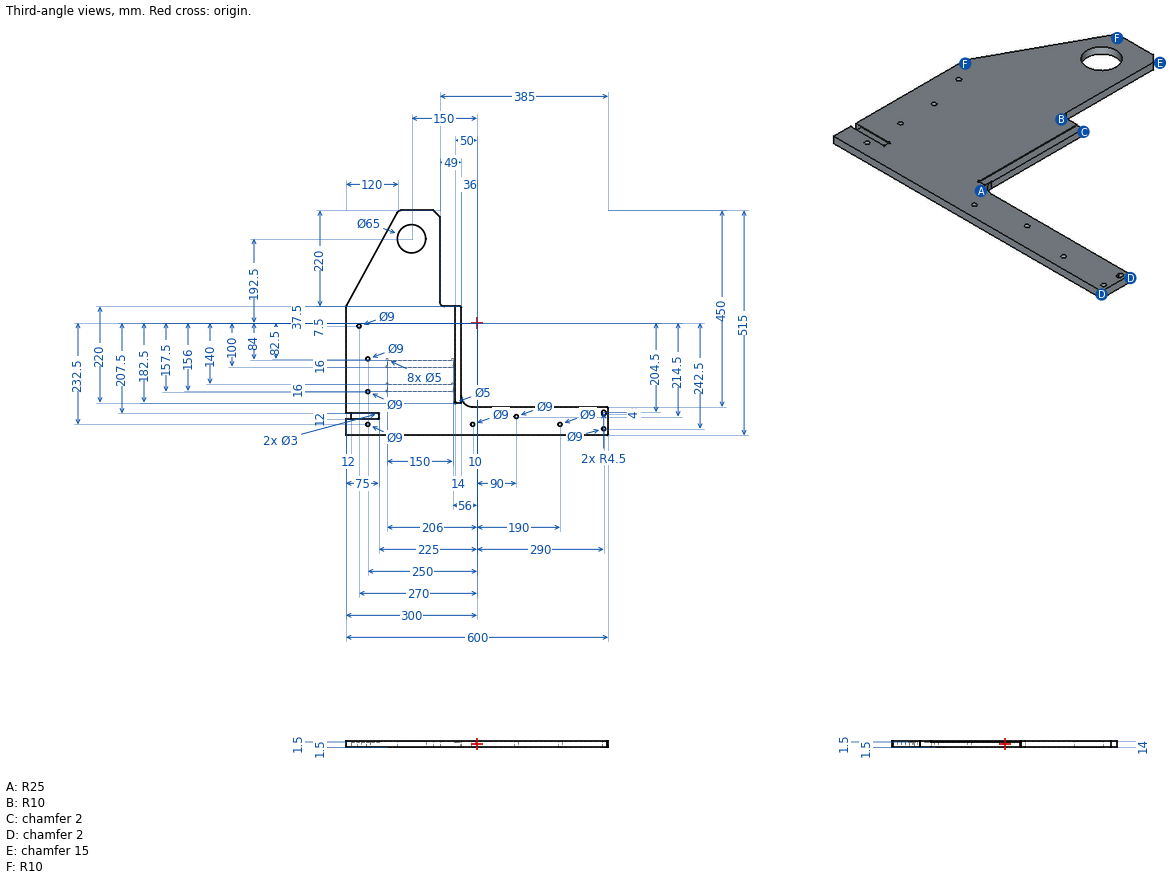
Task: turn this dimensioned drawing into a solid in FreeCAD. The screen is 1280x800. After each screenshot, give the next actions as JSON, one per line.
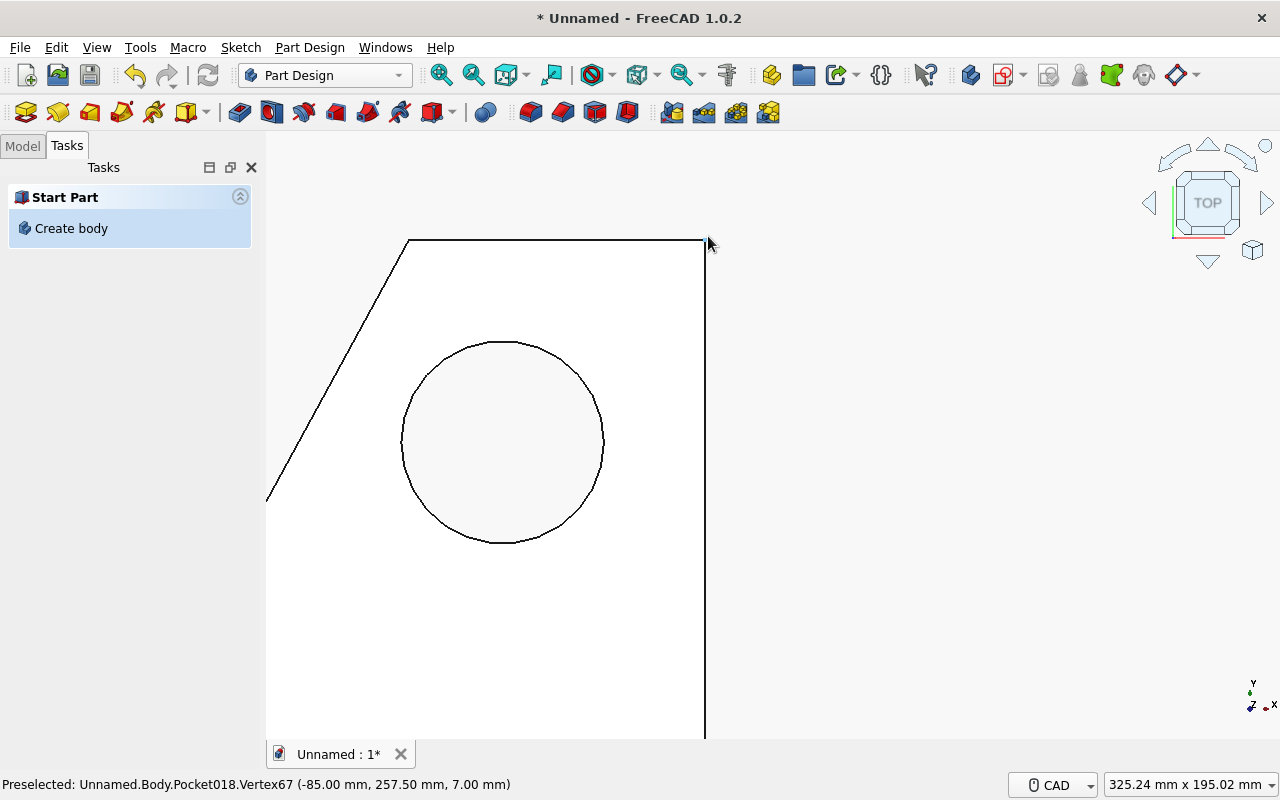
{"action": "left_click", "coordinate": [442, 76]}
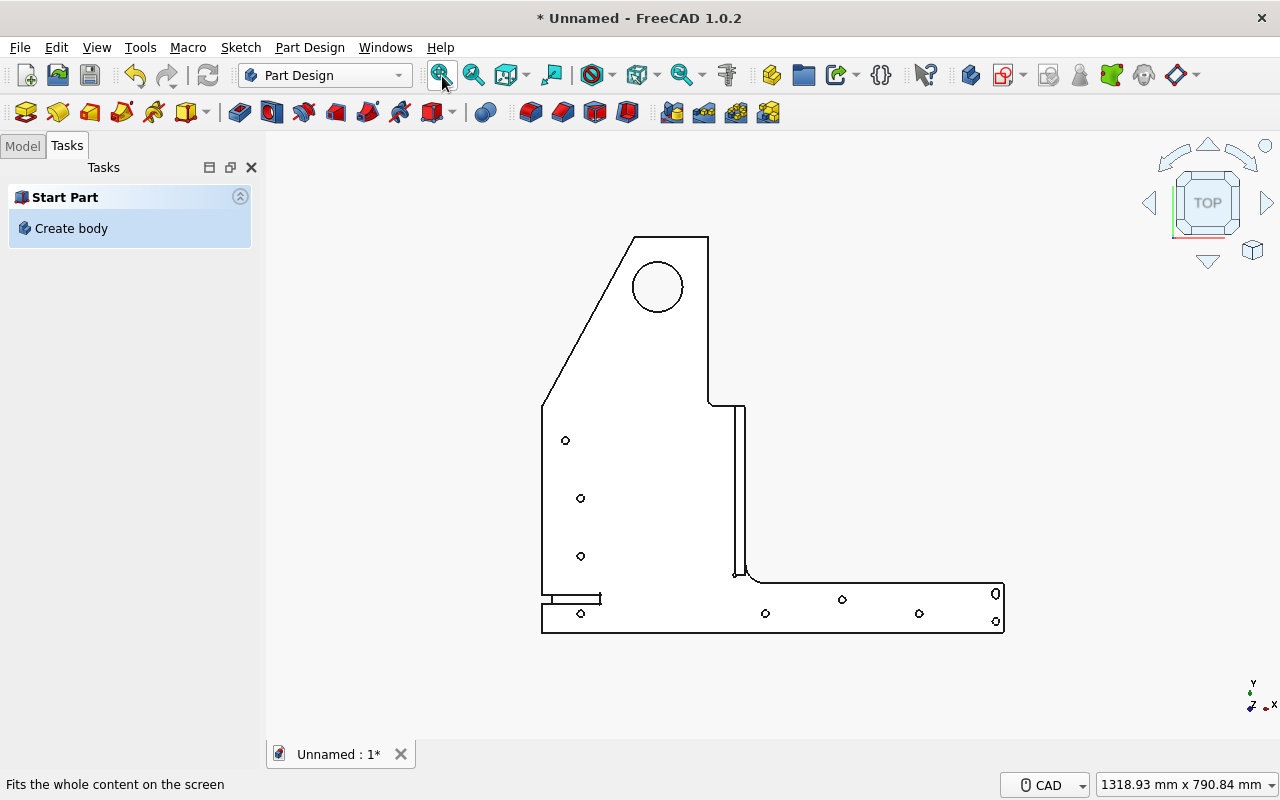
{"action": "key", "text": "0"}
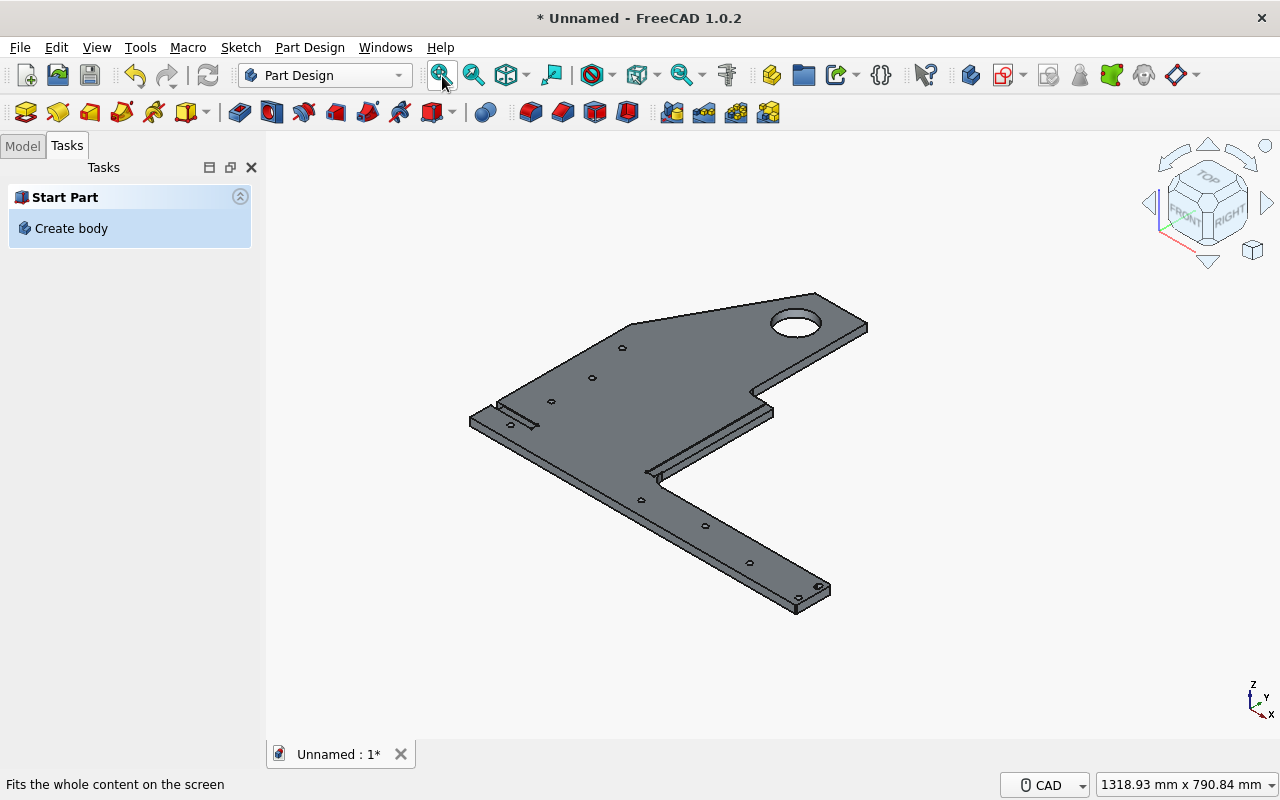
{"action": "scroll", "coordinate": [867, 327], "scroll_direction": "up", "scroll_amount": 7}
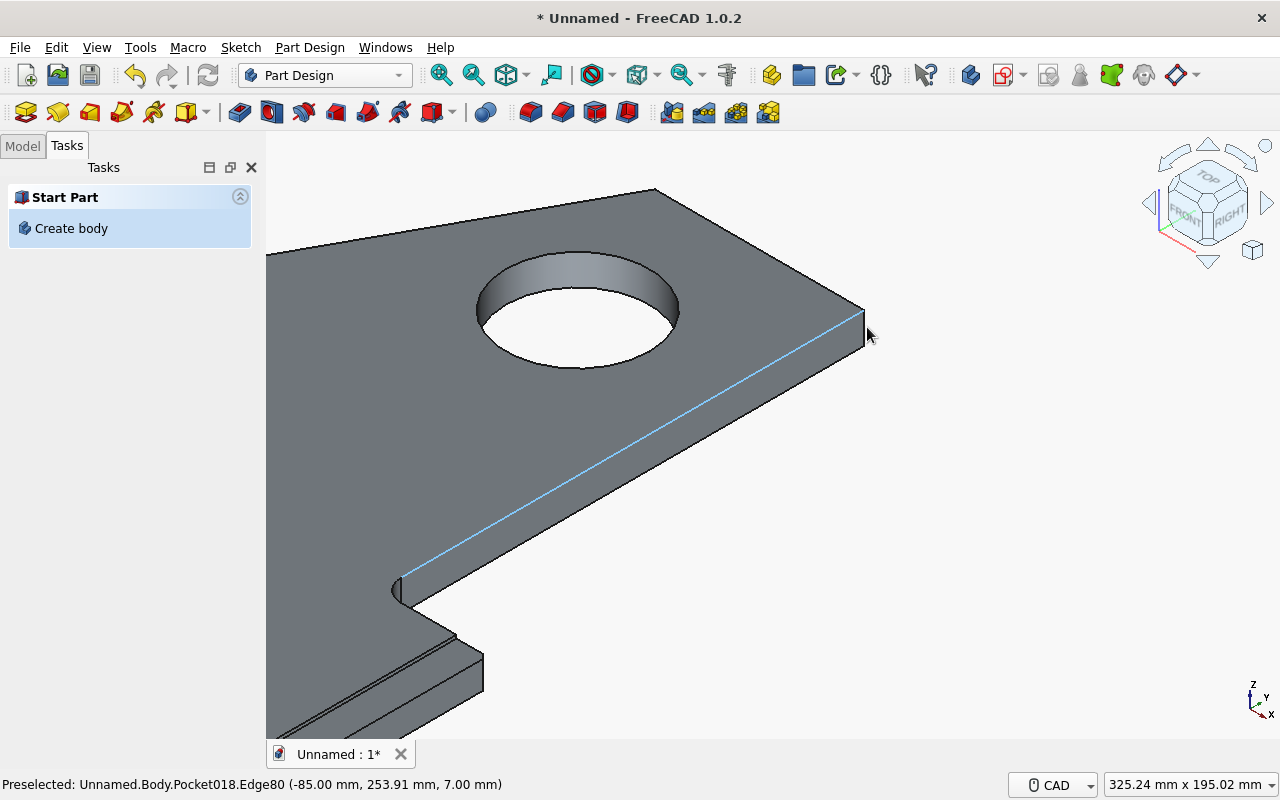
{"action": "left_click", "coordinate": [442, 76]}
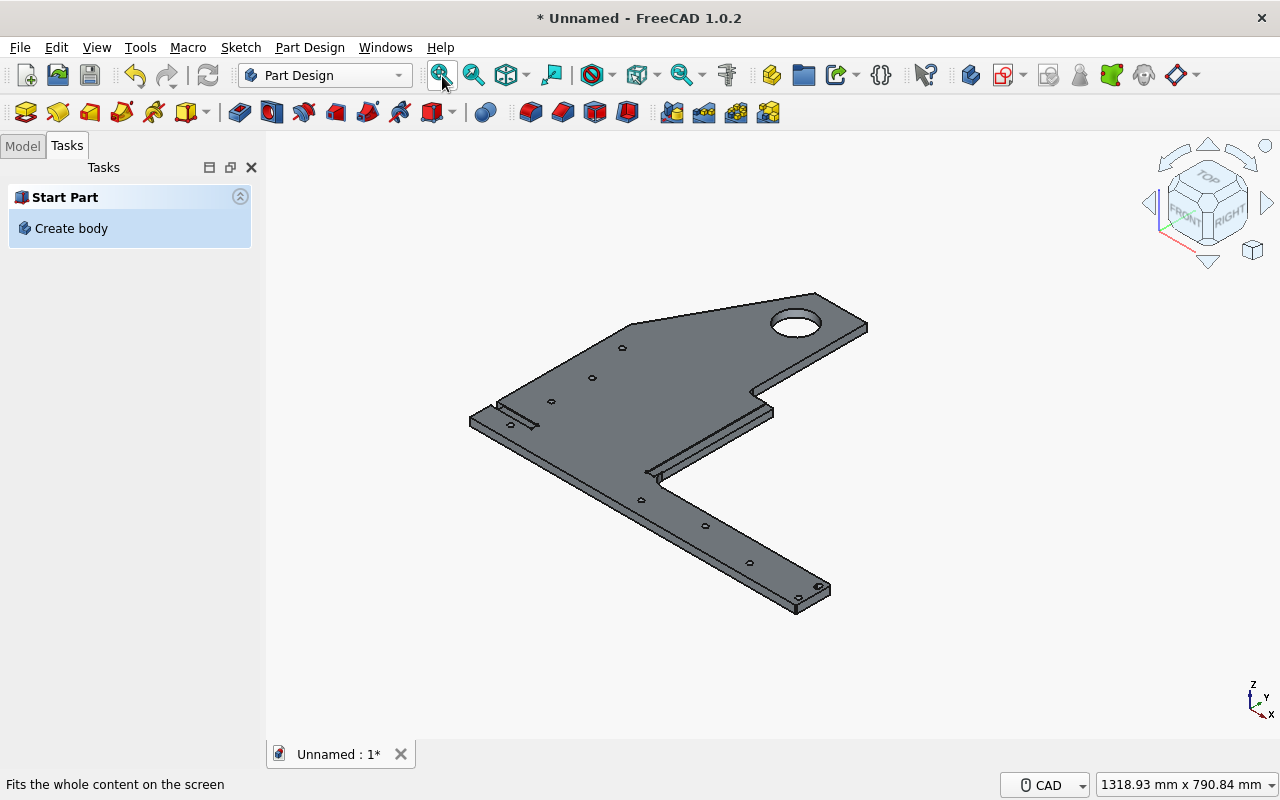
{"action": "key", "text": "1"}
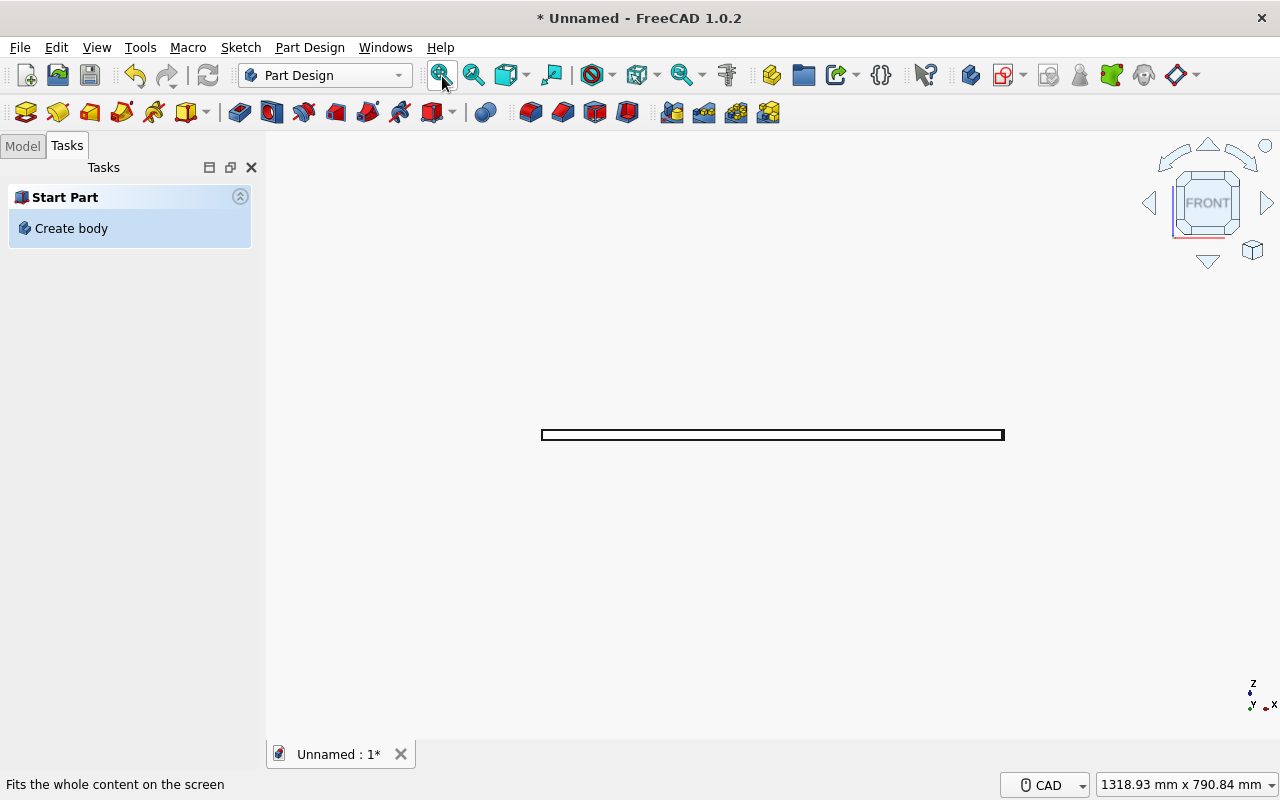
{"action": "scroll", "coordinate": [708, 434], "scroll_direction": "up", "scroll_amount": 7}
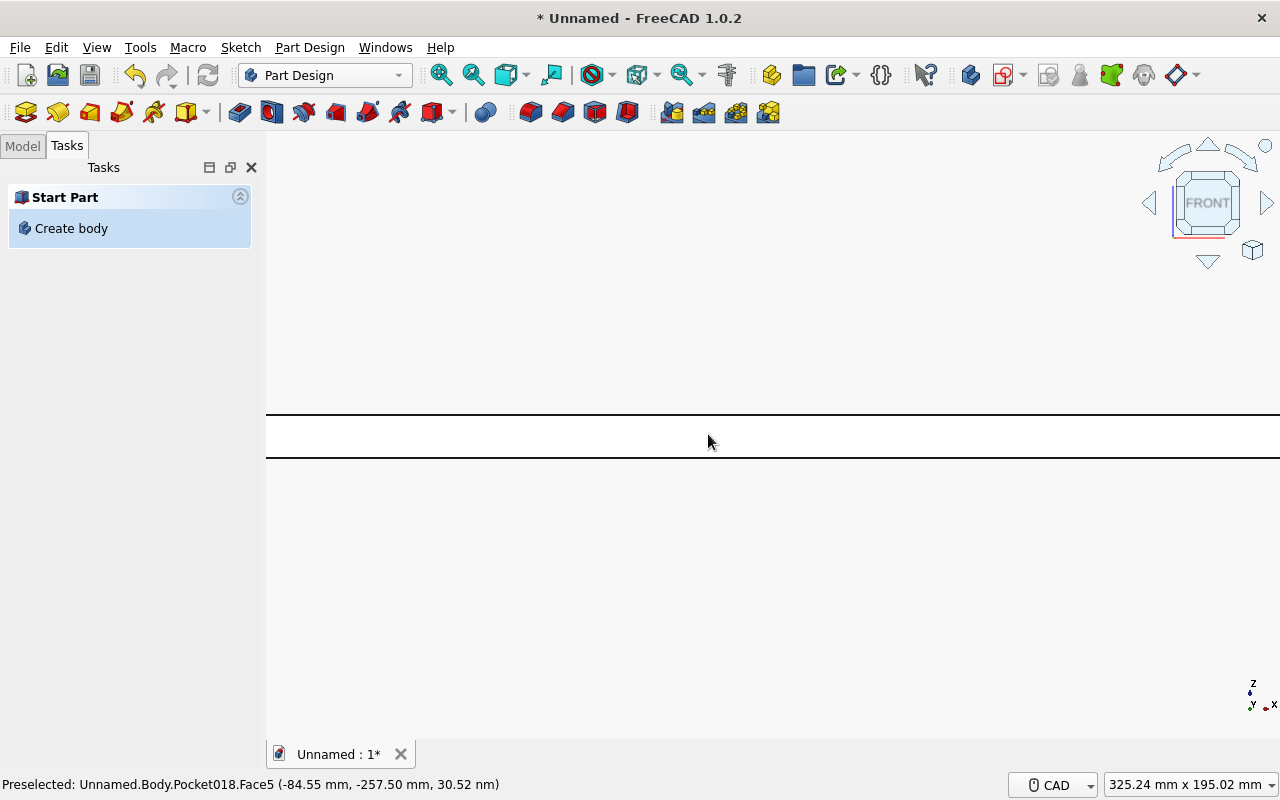
{"action": "left_click", "coordinate": [442, 76]}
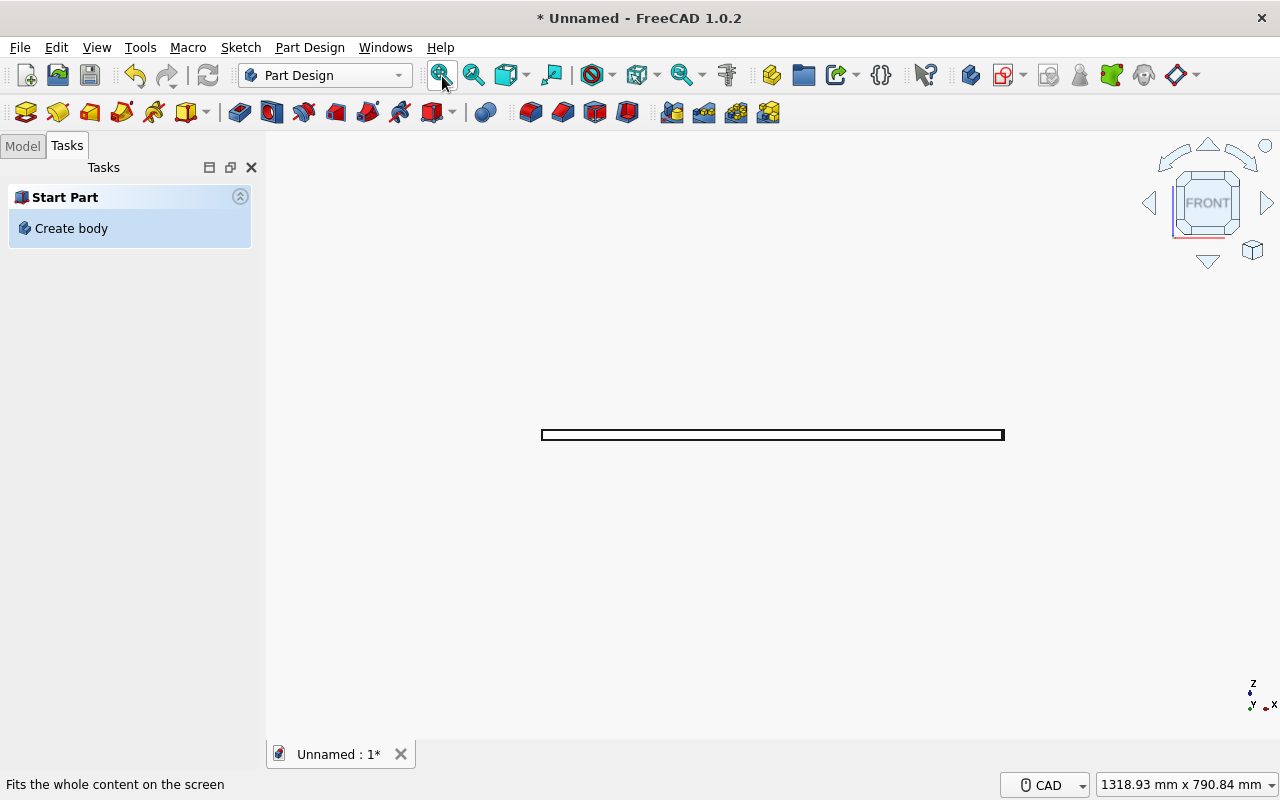
{"action": "key", "text": "3"}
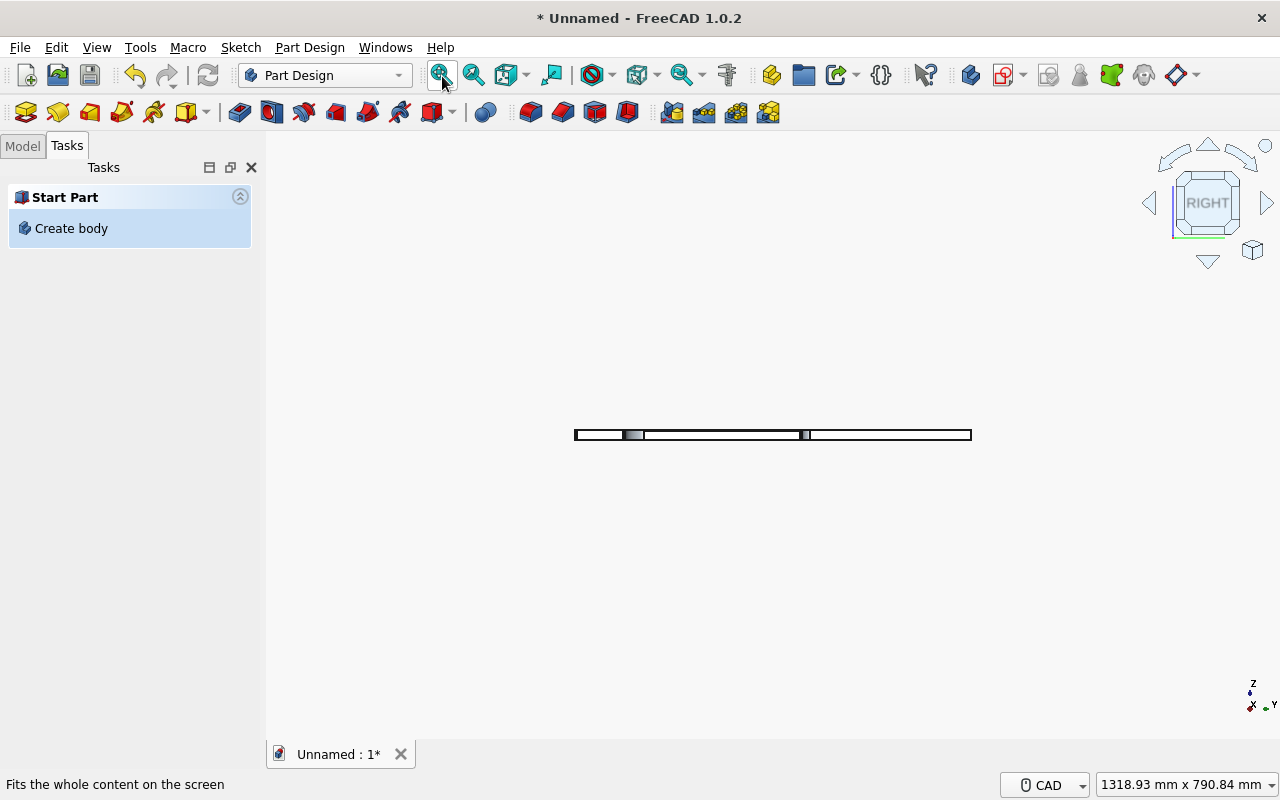
{"action": "left_click", "coordinate": [442, 76]}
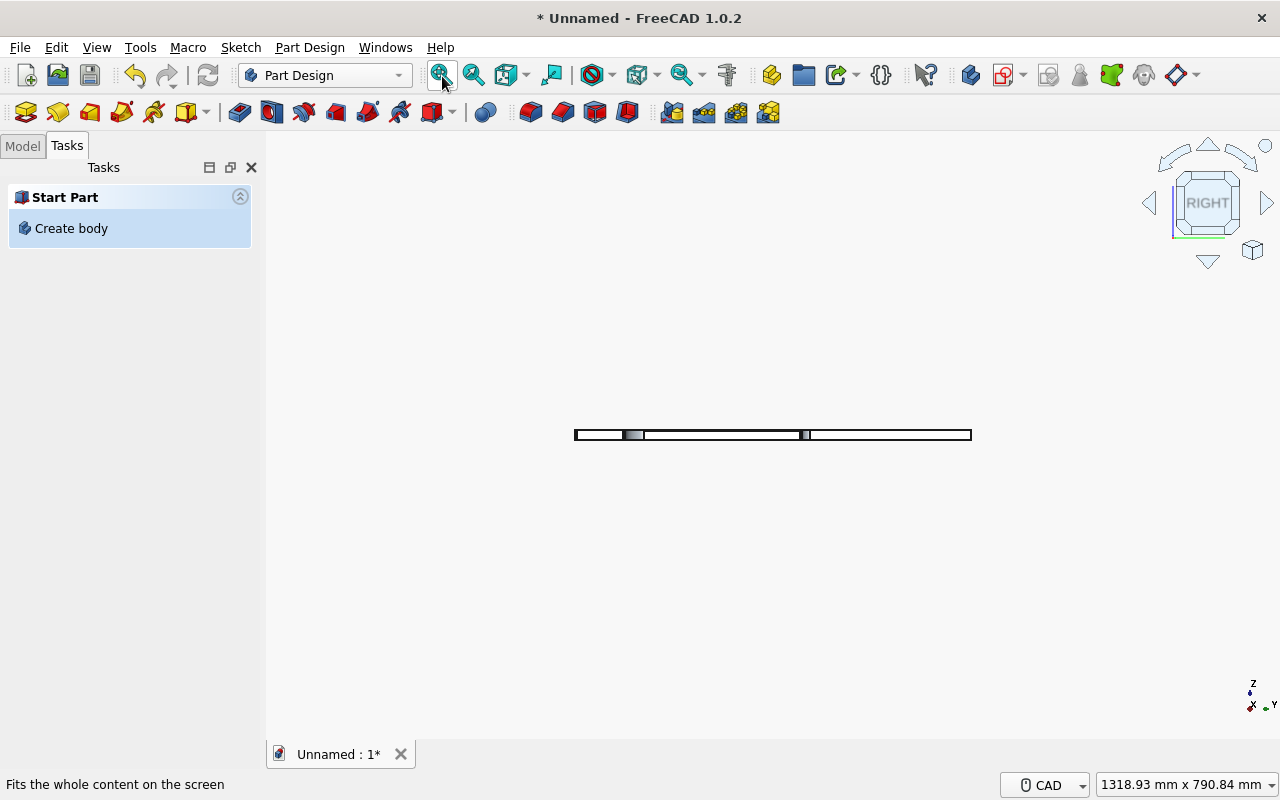
{"action": "scroll", "coordinate": [971, 434], "scroll_direction": "up", "scroll_amount": 7}